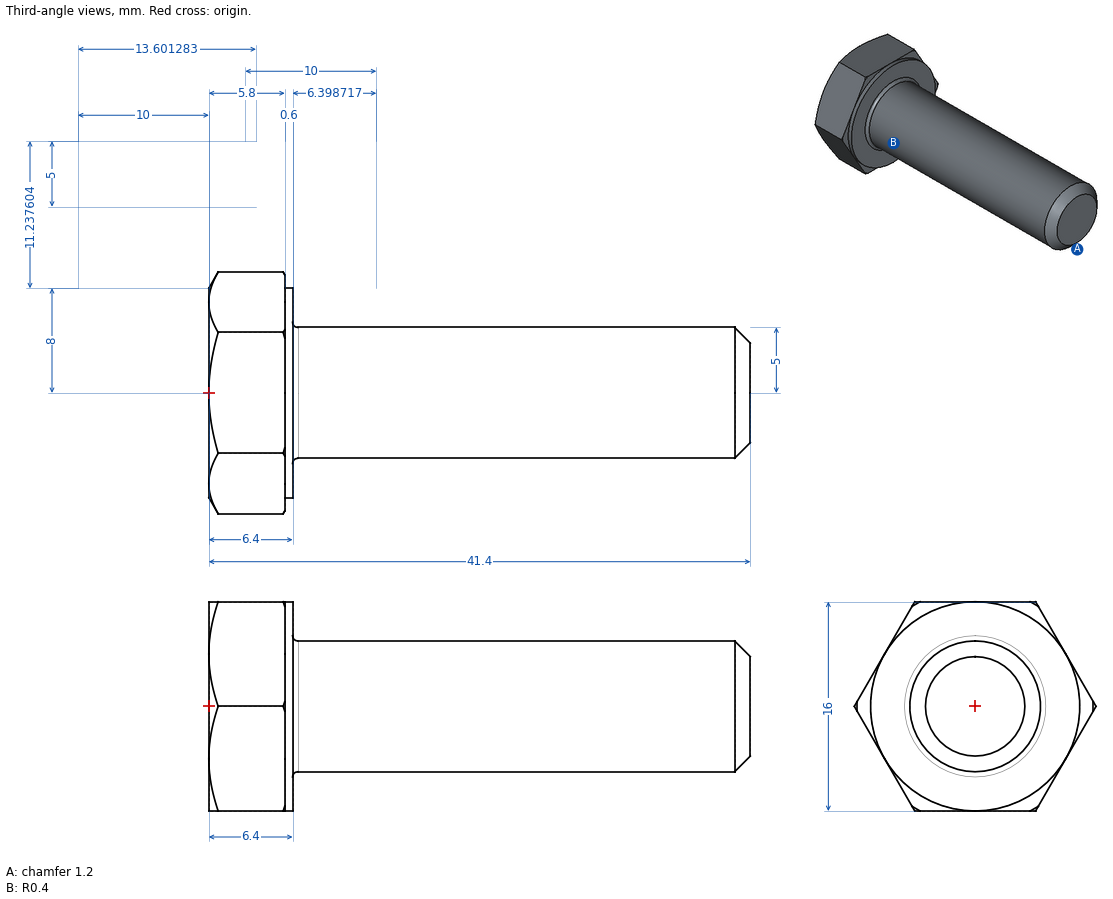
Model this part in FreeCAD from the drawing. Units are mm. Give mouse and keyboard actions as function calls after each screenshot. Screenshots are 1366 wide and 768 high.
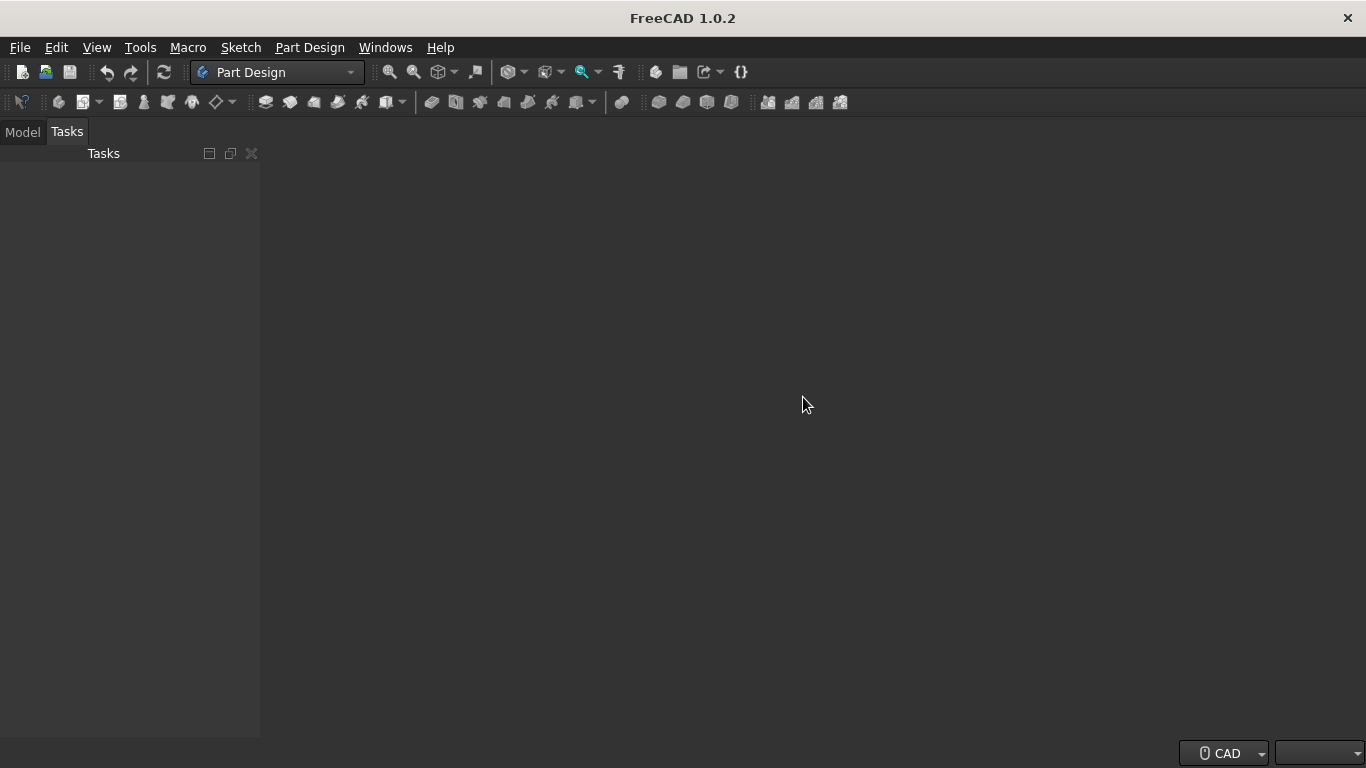
key(ctrl+n)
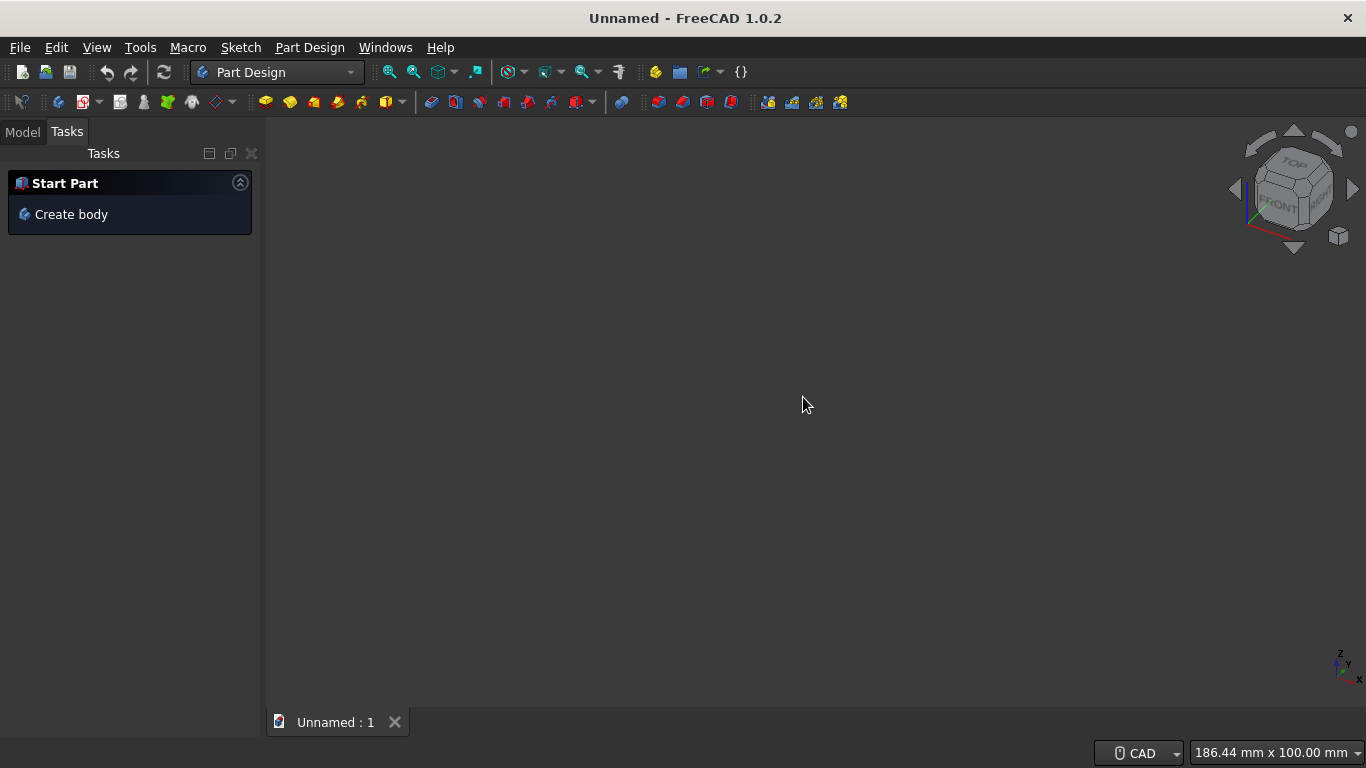
click(84, 102)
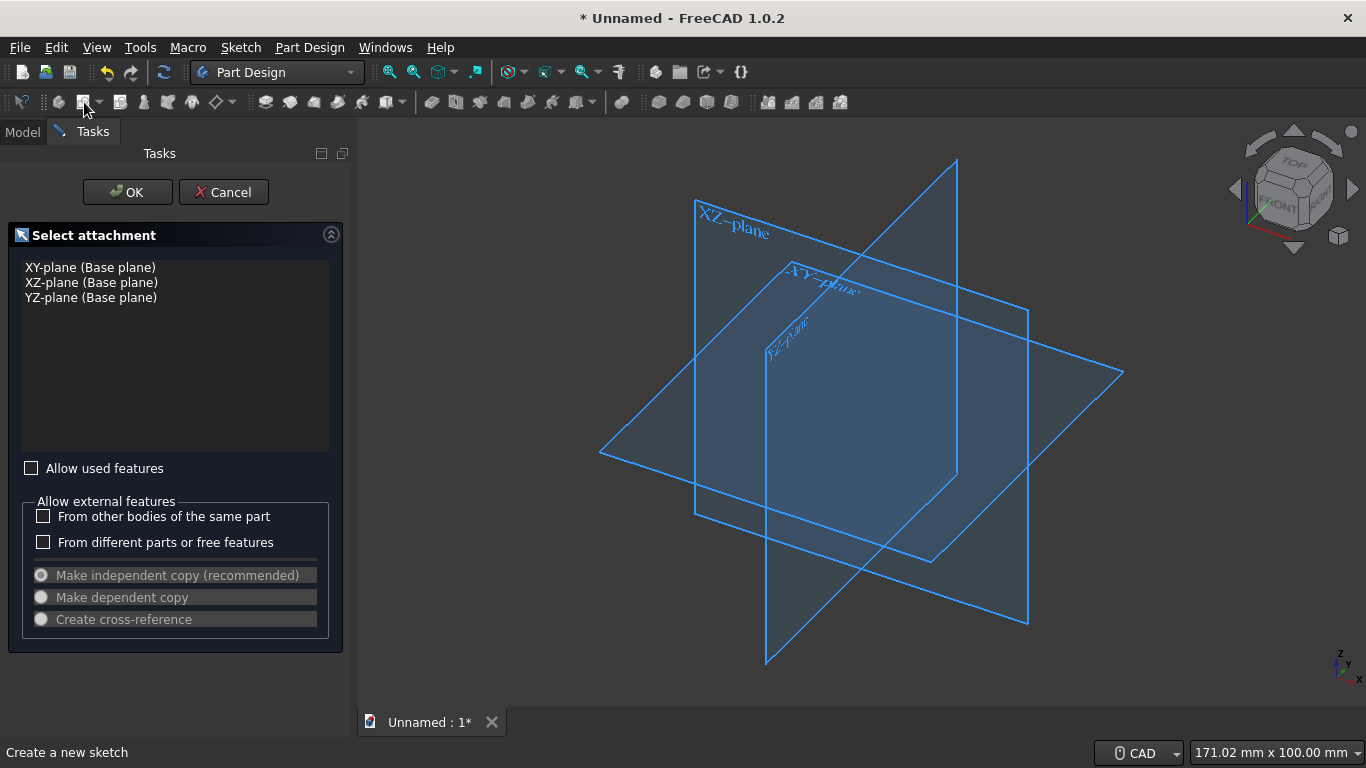
click(82, 298)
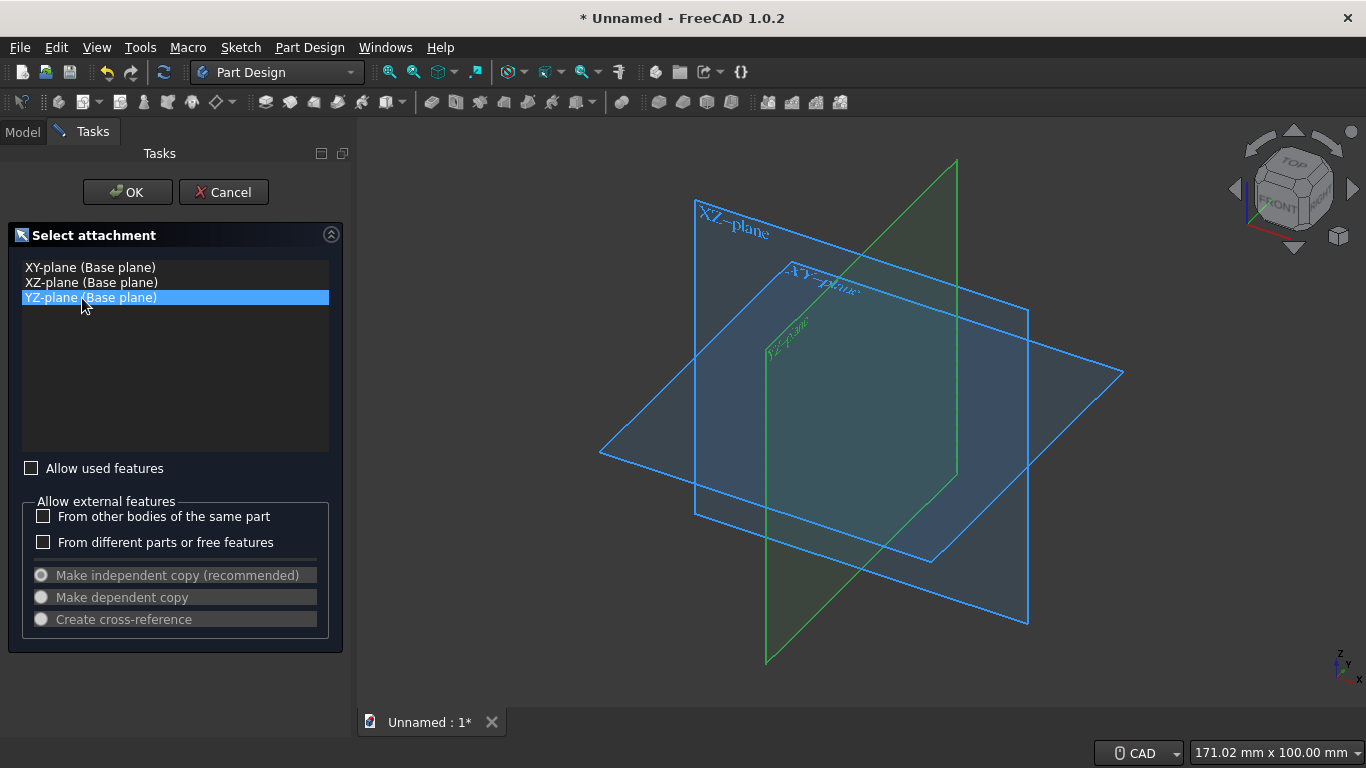
click(128, 192)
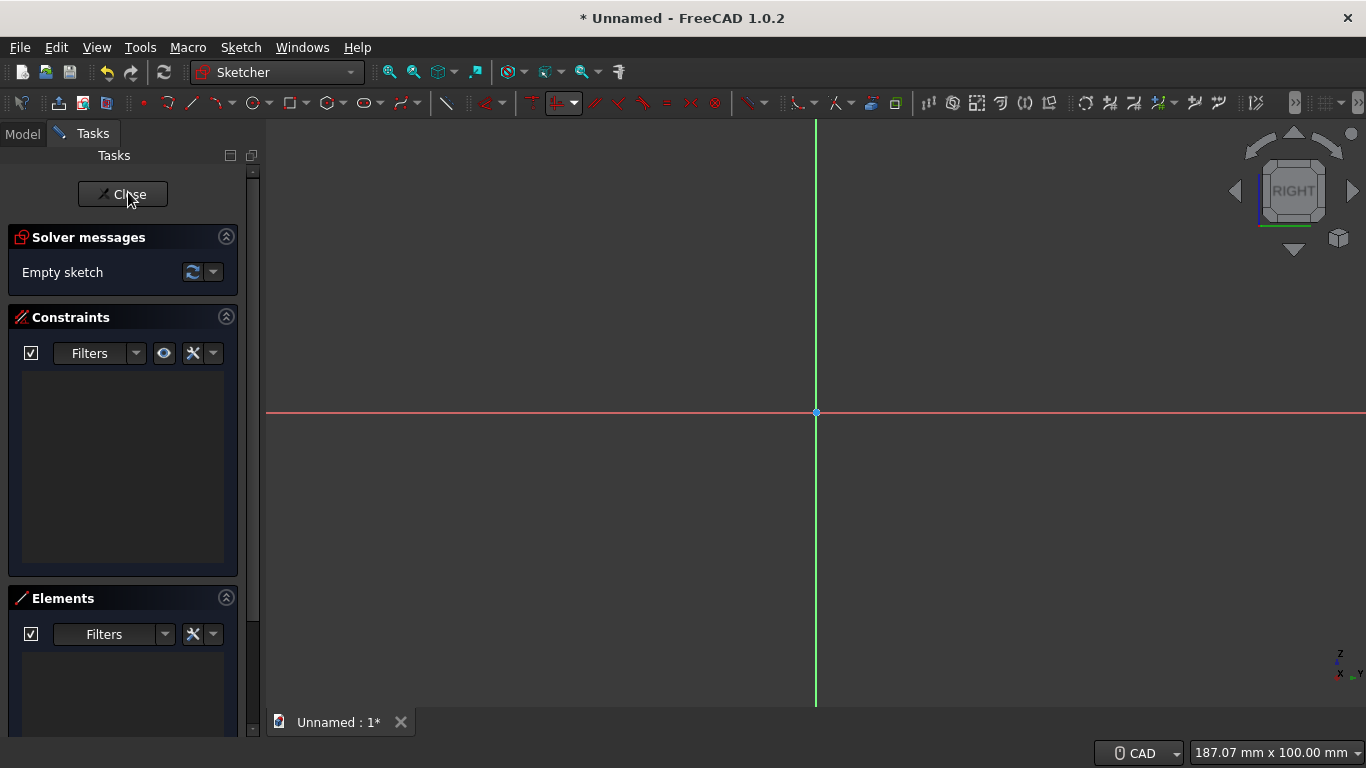
scroll(838, 413, up, 7)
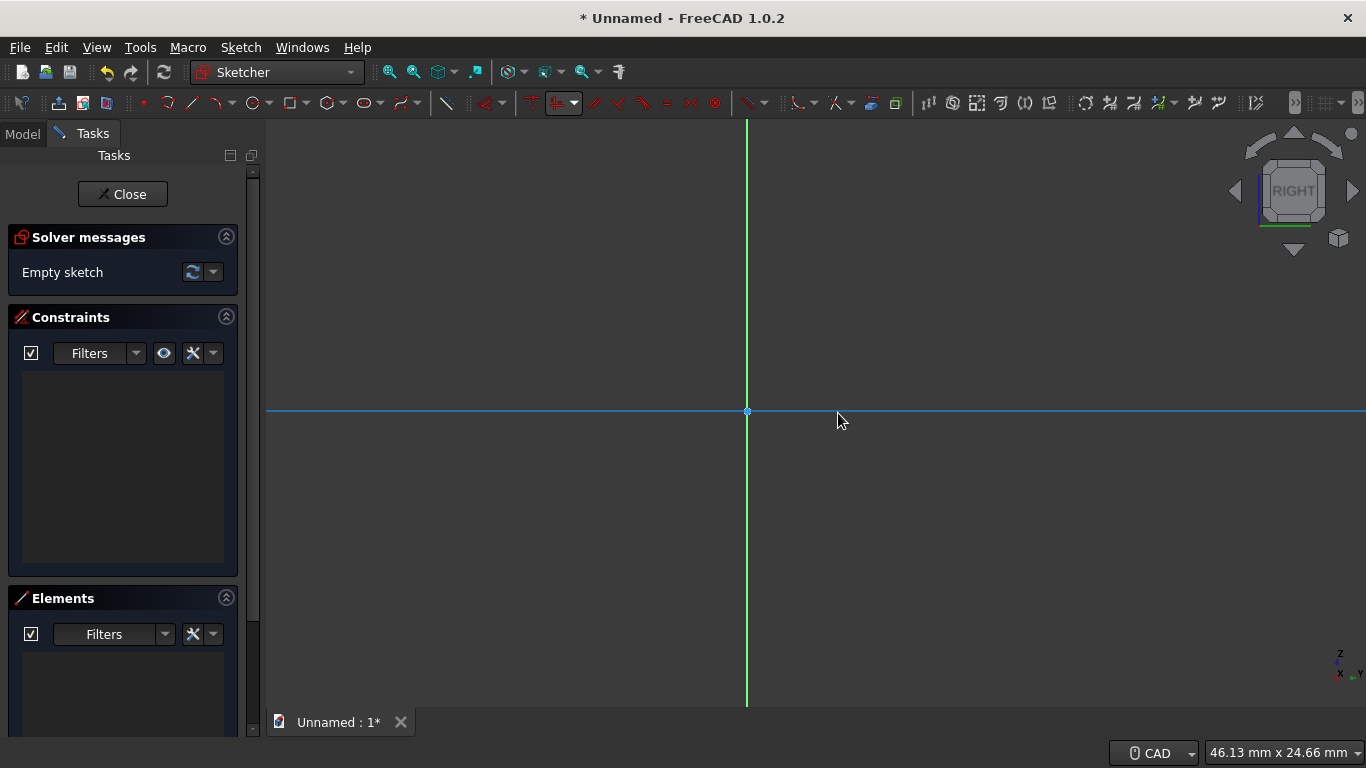
click(328, 104)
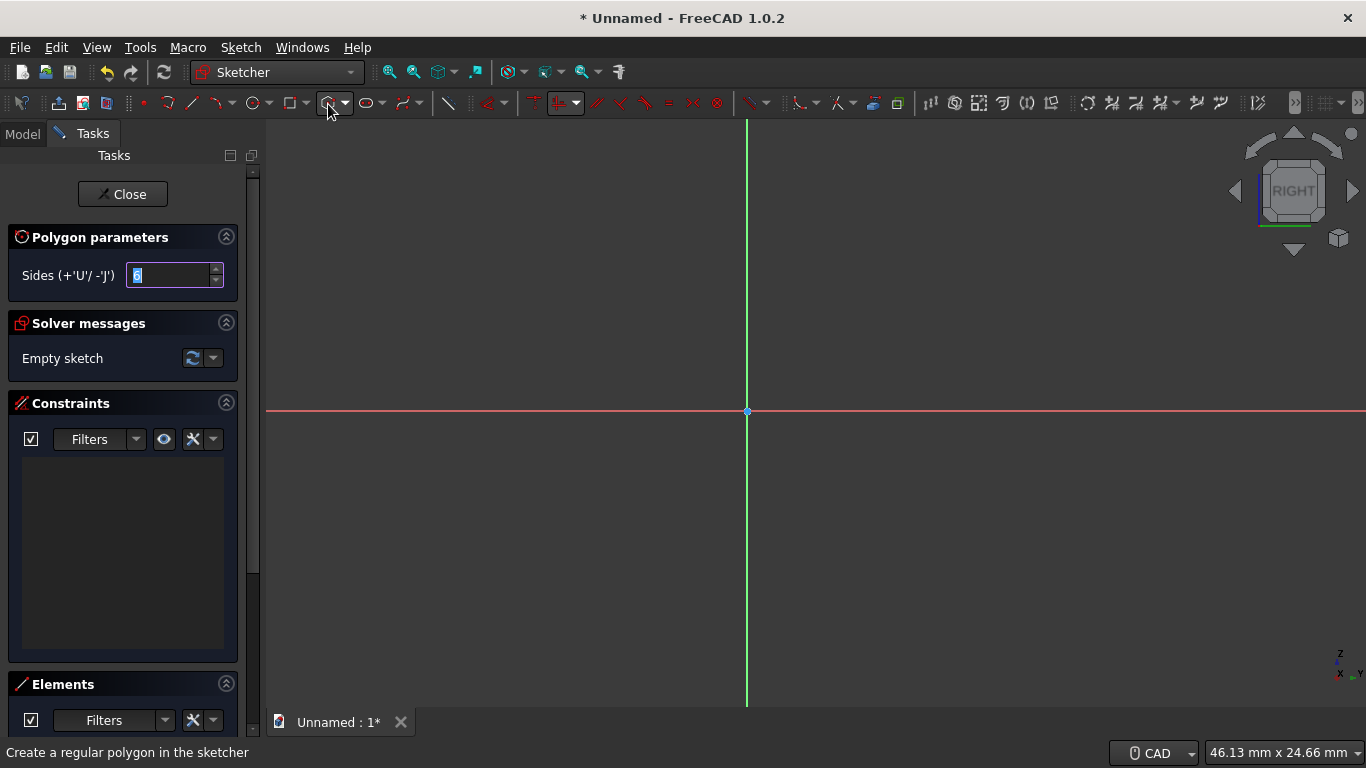
click(747, 411)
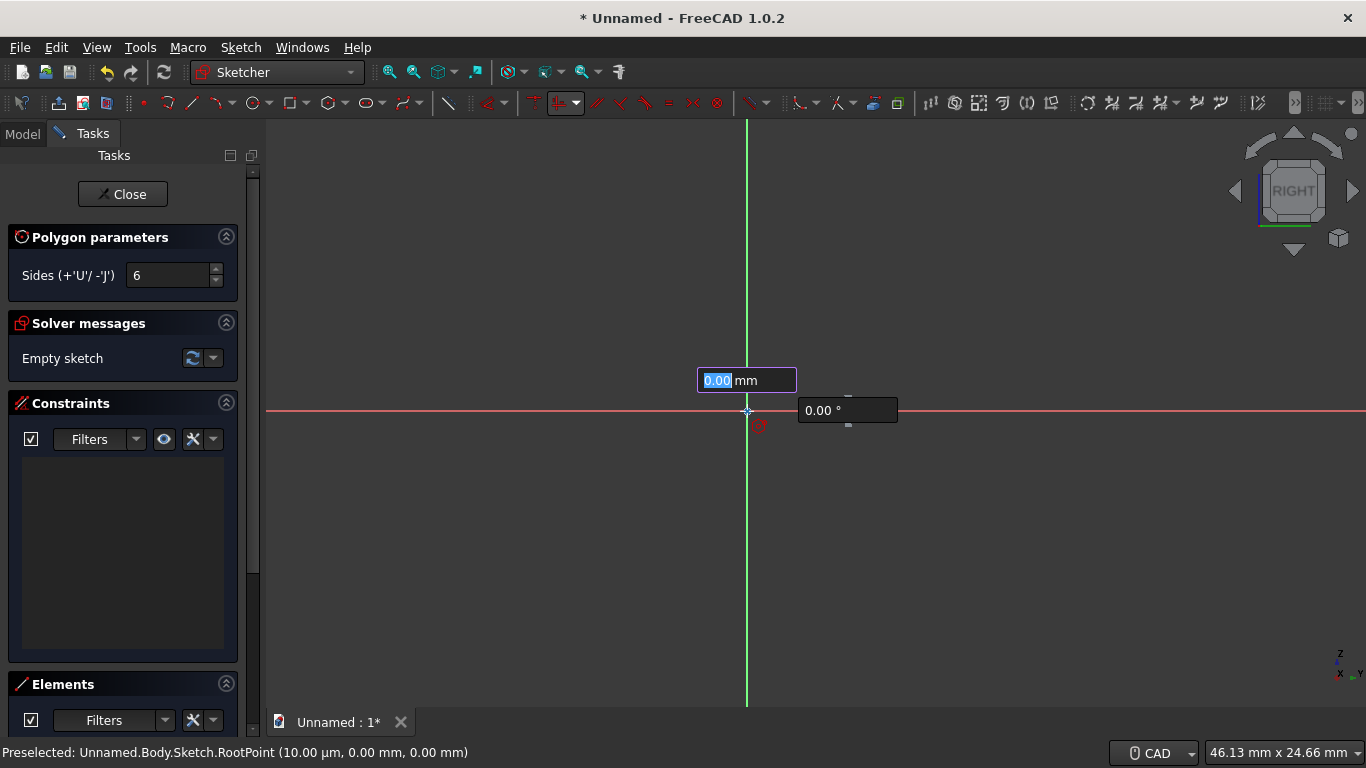
click(967, 411)
right_click(967, 411)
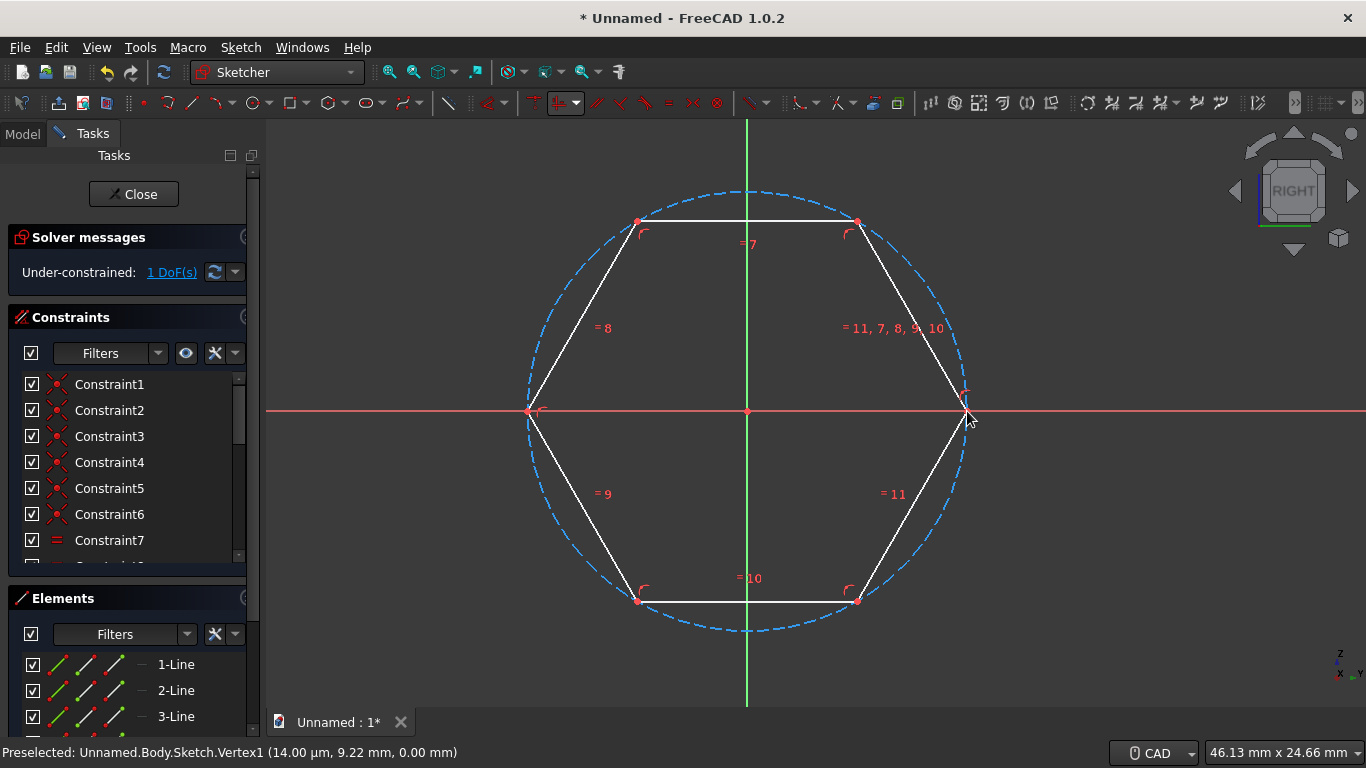
click(488, 104)